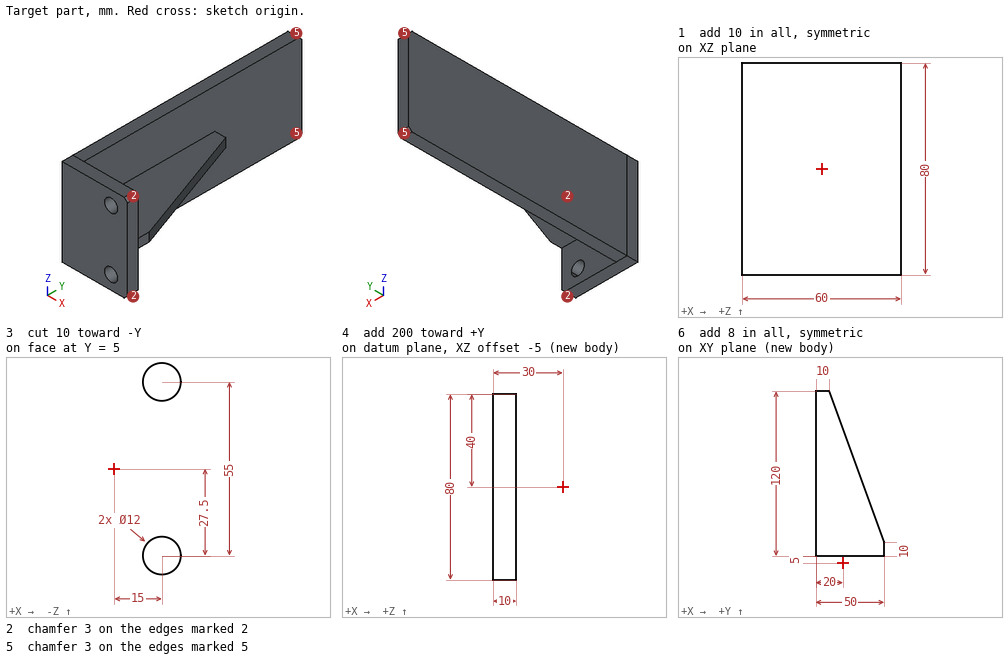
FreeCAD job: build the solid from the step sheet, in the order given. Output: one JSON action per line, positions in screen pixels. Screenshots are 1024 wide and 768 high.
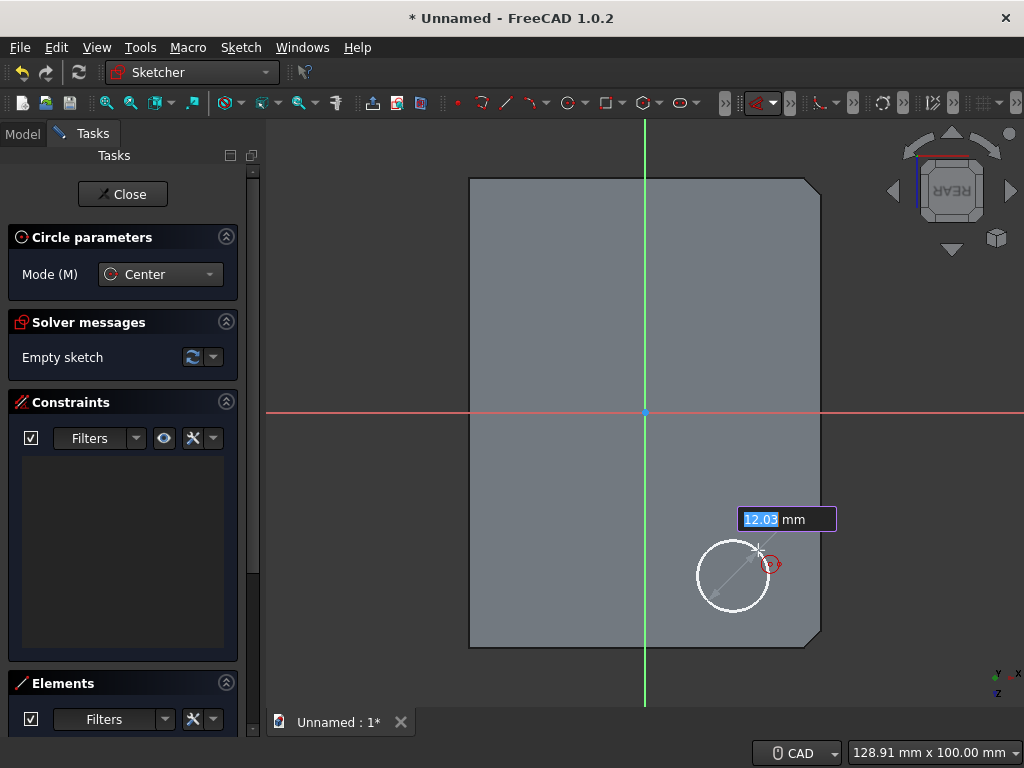
{"action": "type", "text": "12"}
{"action": "key", "text": "Return"}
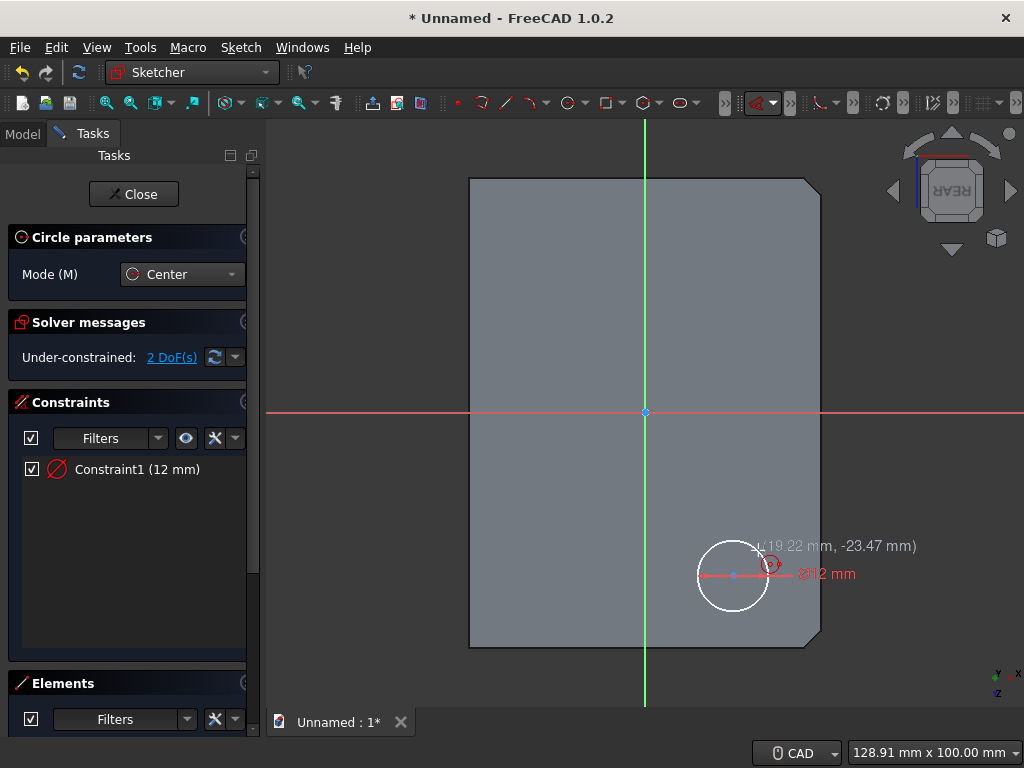
{"action": "left_click", "coordinate": [733, 251]}
{"action": "mouse_move", "coordinate": [758, 226]}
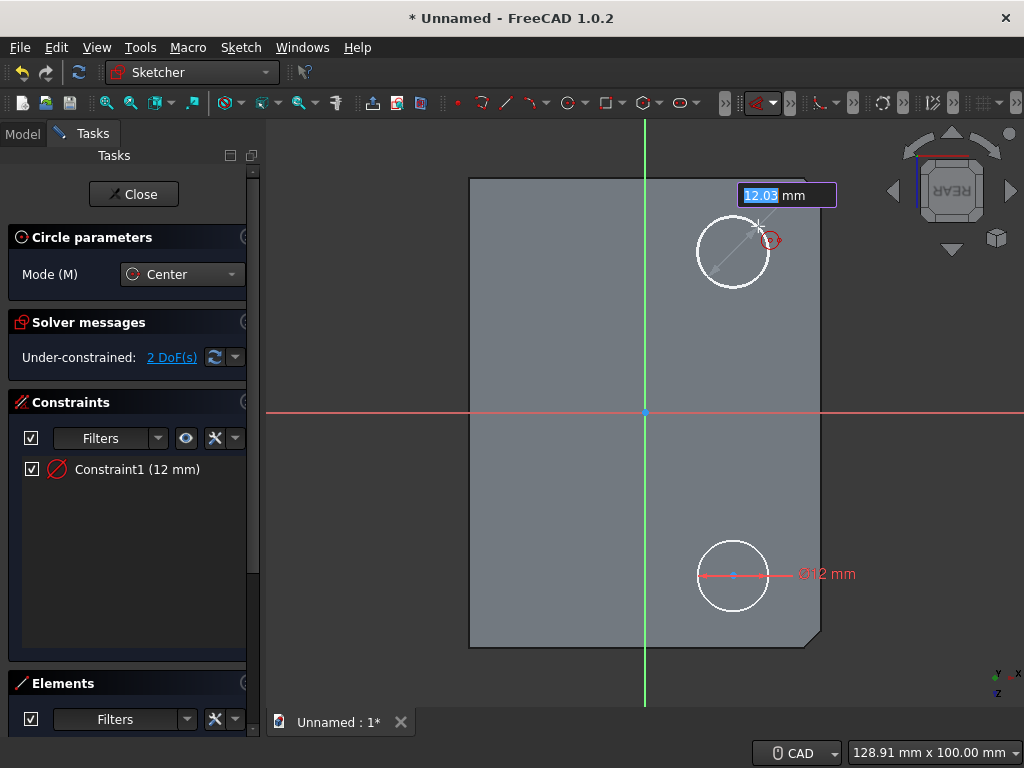
{"action": "type", "text": "12"}
{"action": "key", "text": "Return"}
{"action": "key", "text": "Escape"}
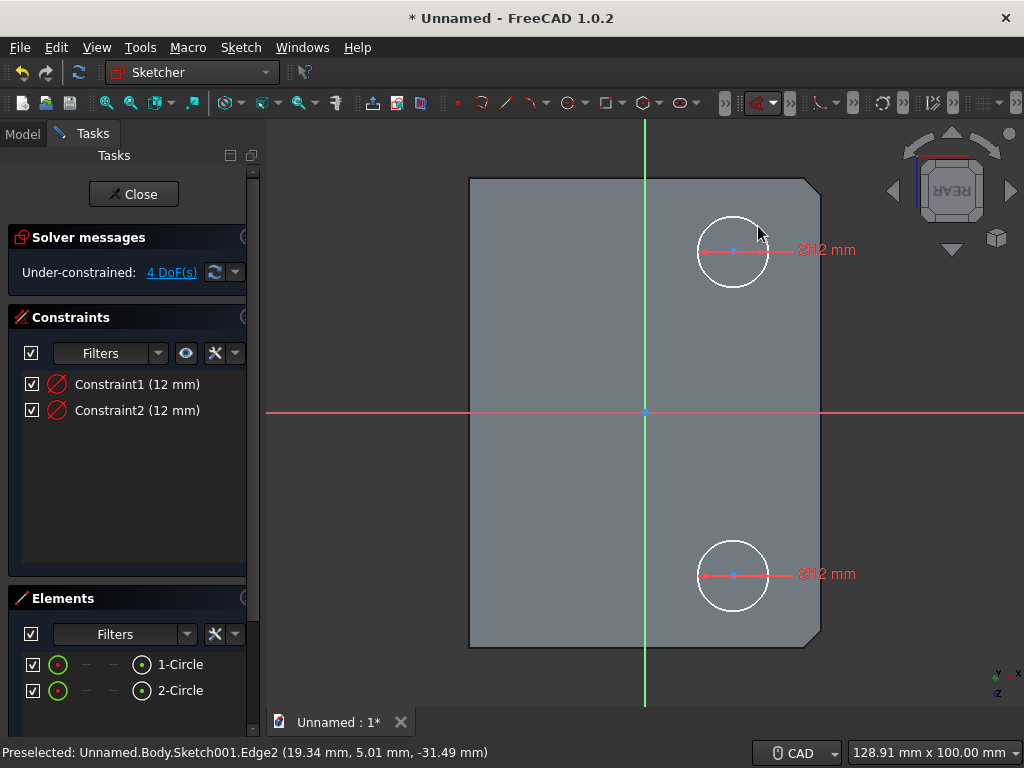
{"action": "left_click", "coordinate": [733, 576]}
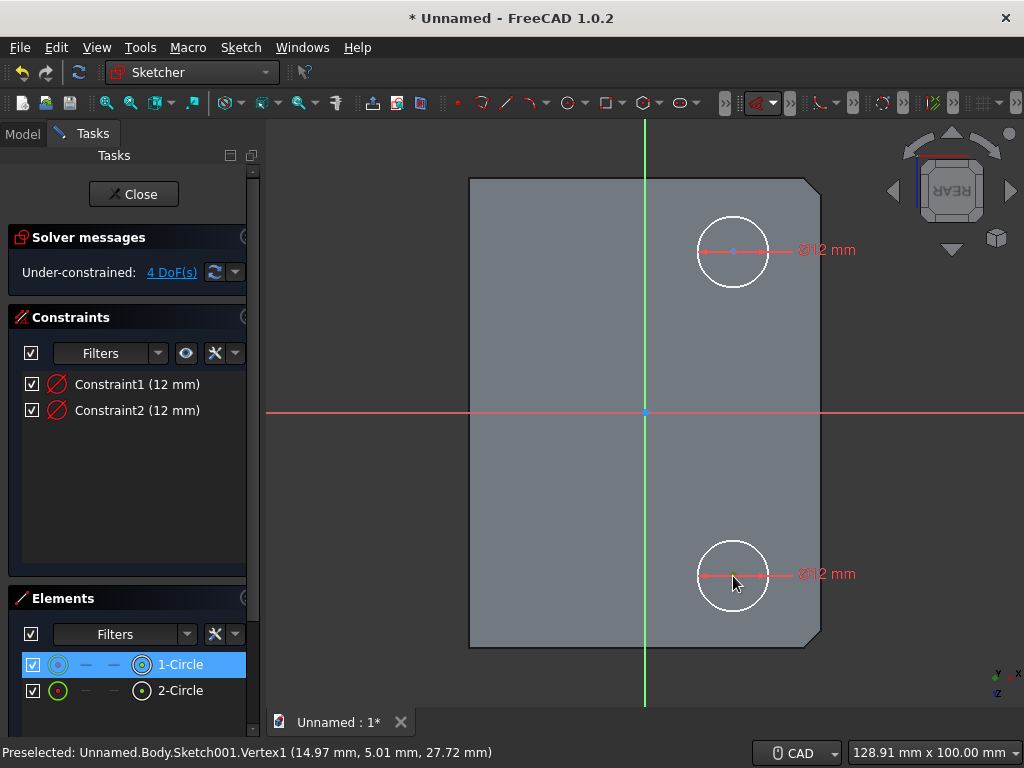
{"action": "left_click", "coordinate": [733, 252]}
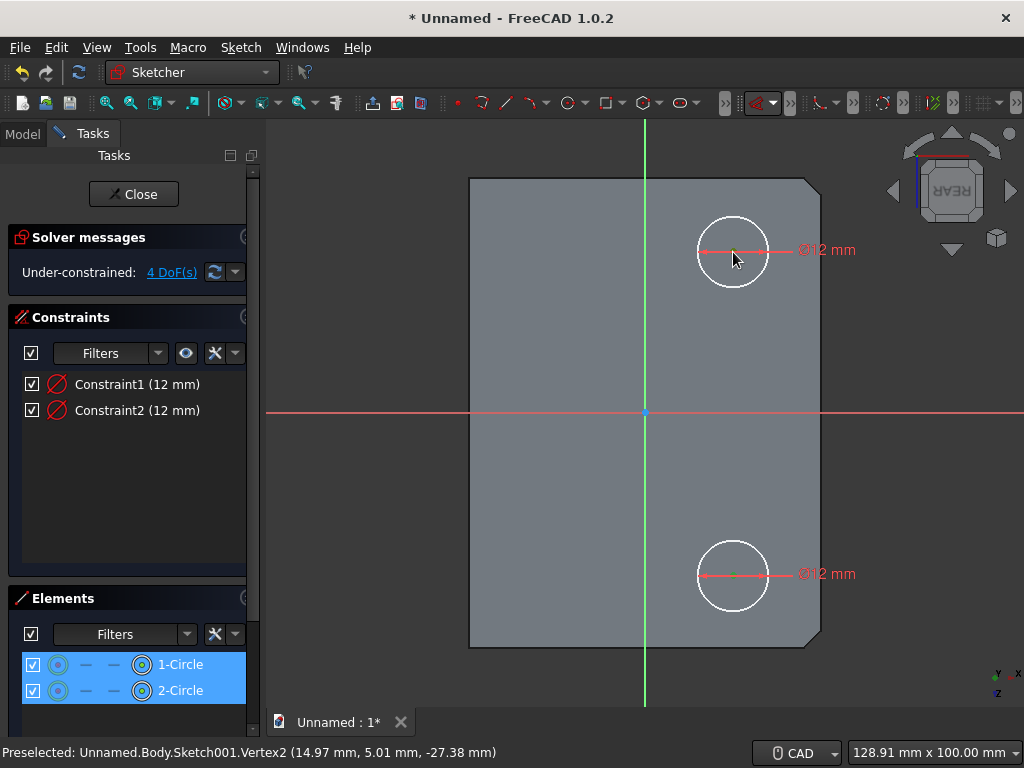
{"action": "key", "text": "v"}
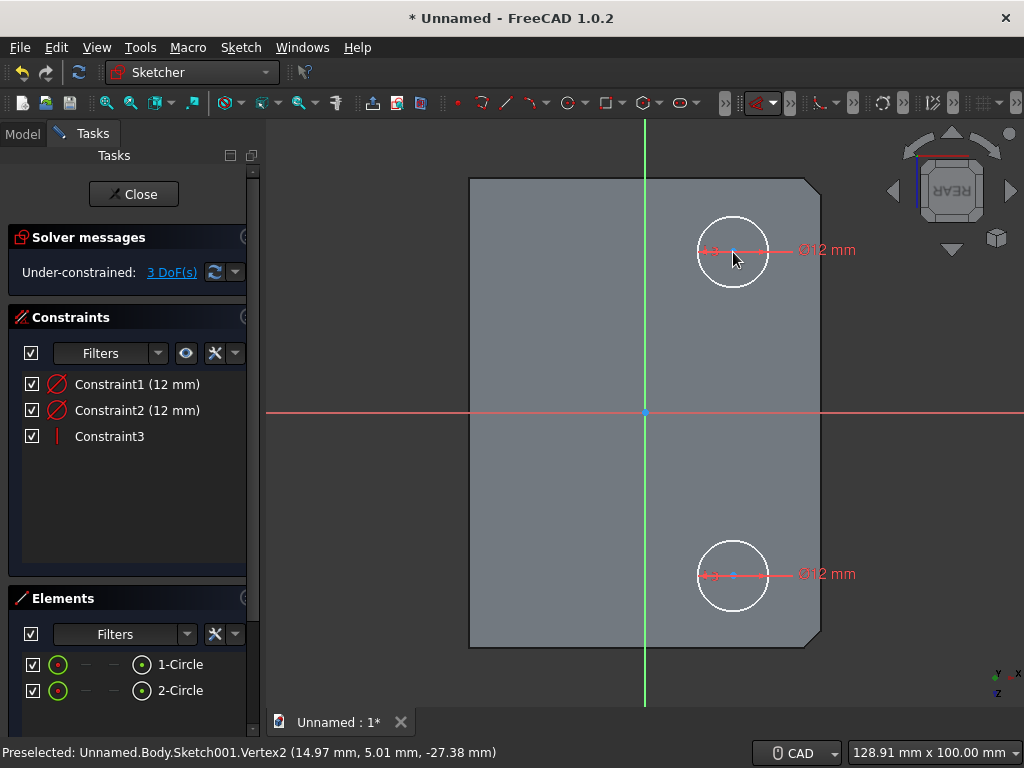
{"action": "left_click", "coordinate": [733, 576]}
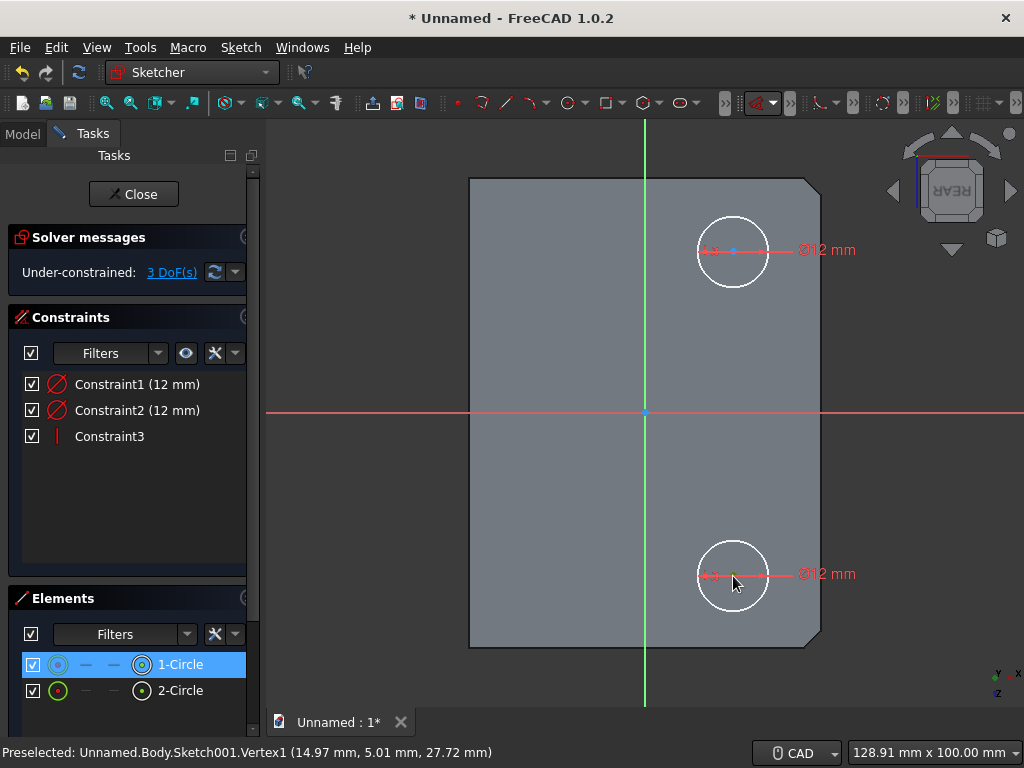
{"action": "left_click", "coordinate": [776, 104]}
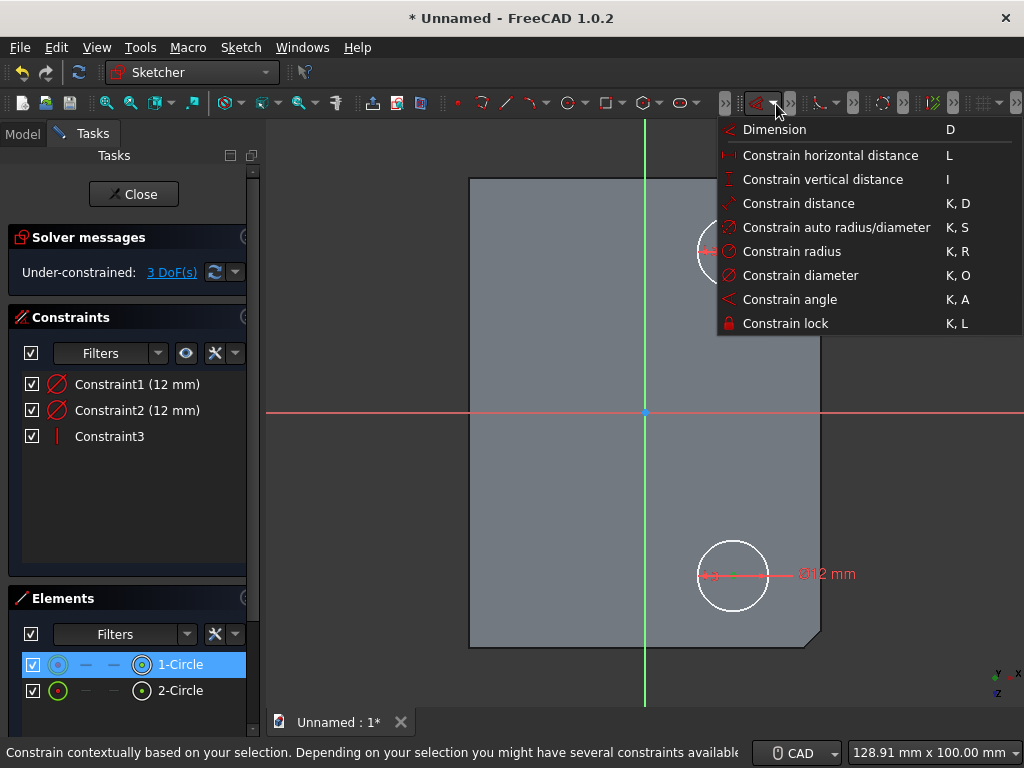
{"action": "left_click", "coordinate": [870, 155]}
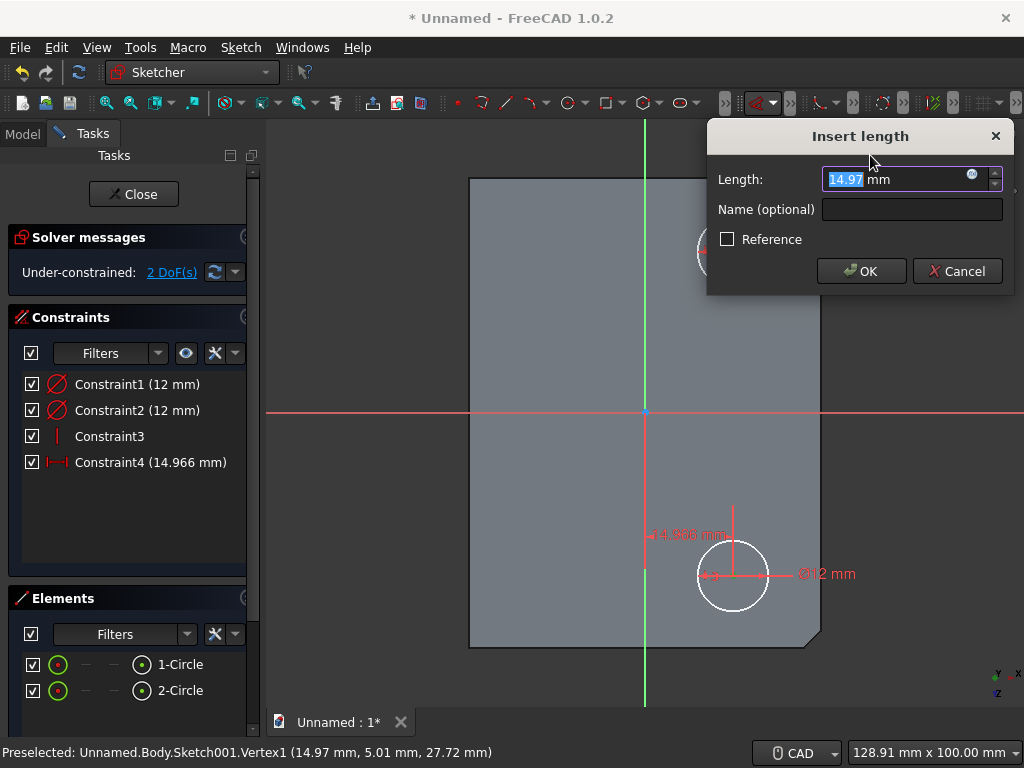
{"action": "type", "text": "15"}
{"action": "key", "text": "Return"}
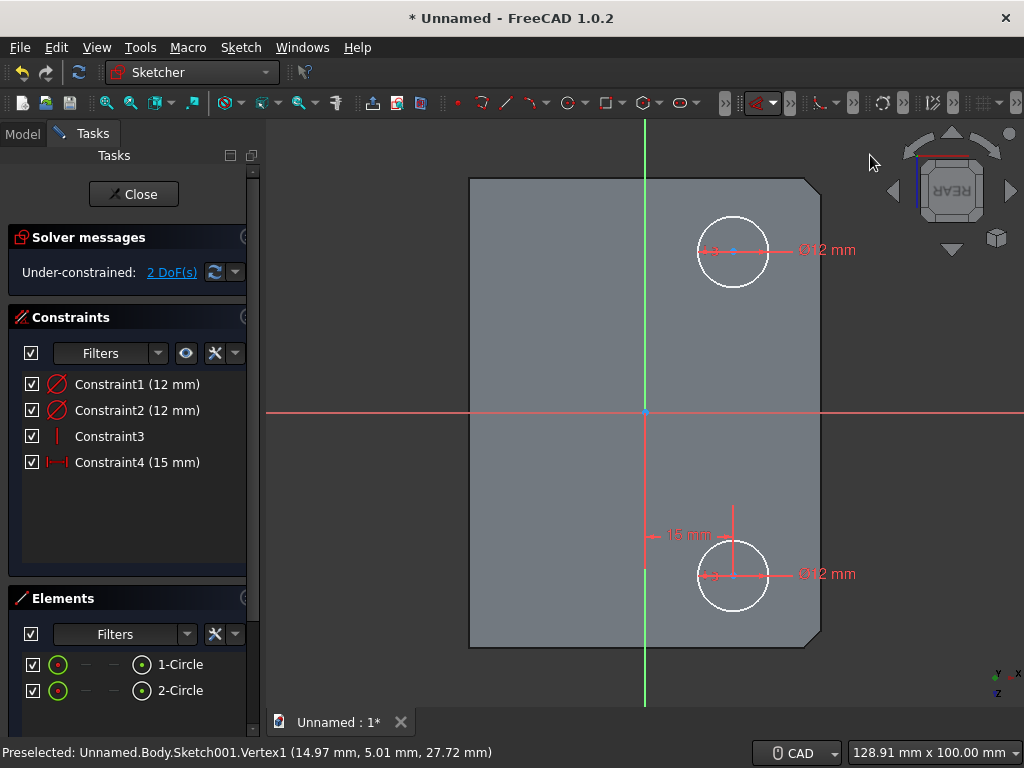
{"action": "left_click", "coordinate": [733, 576]}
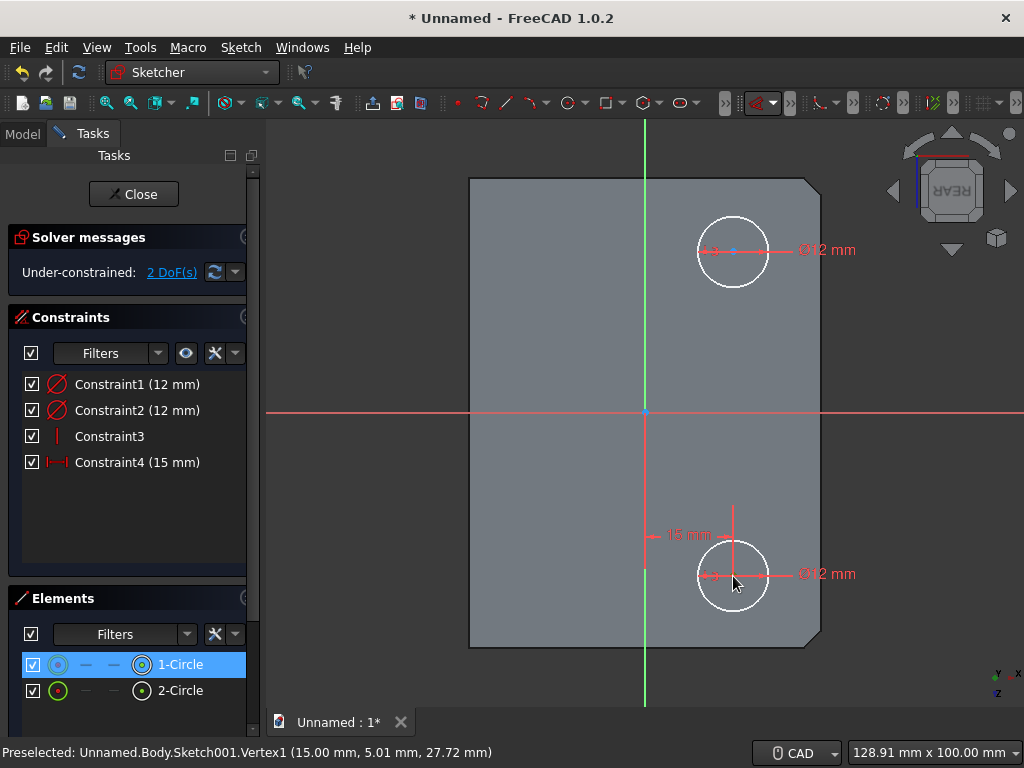
{"action": "left_click", "coordinate": [733, 252]}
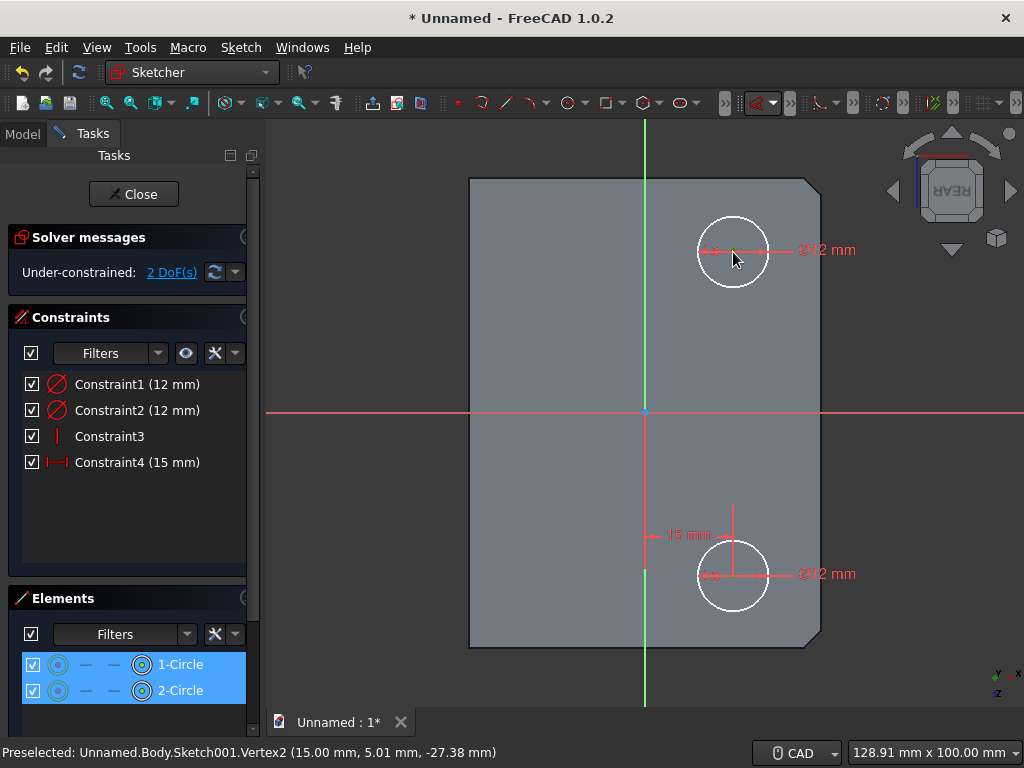
{"action": "left_click", "coordinate": [776, 104]}